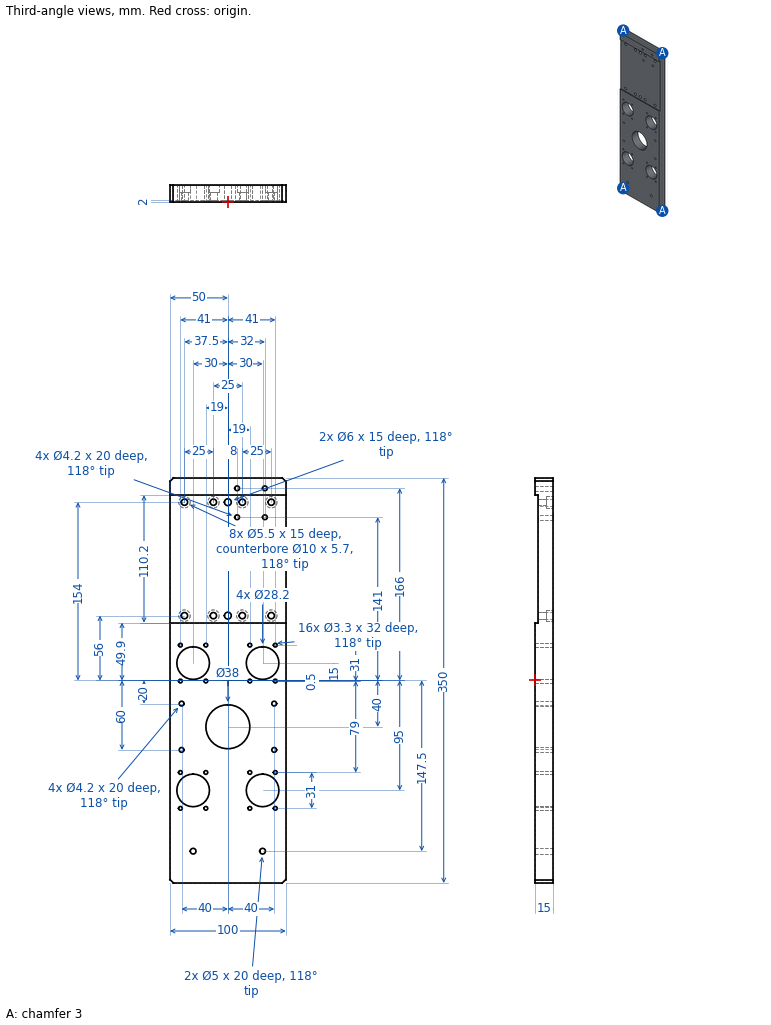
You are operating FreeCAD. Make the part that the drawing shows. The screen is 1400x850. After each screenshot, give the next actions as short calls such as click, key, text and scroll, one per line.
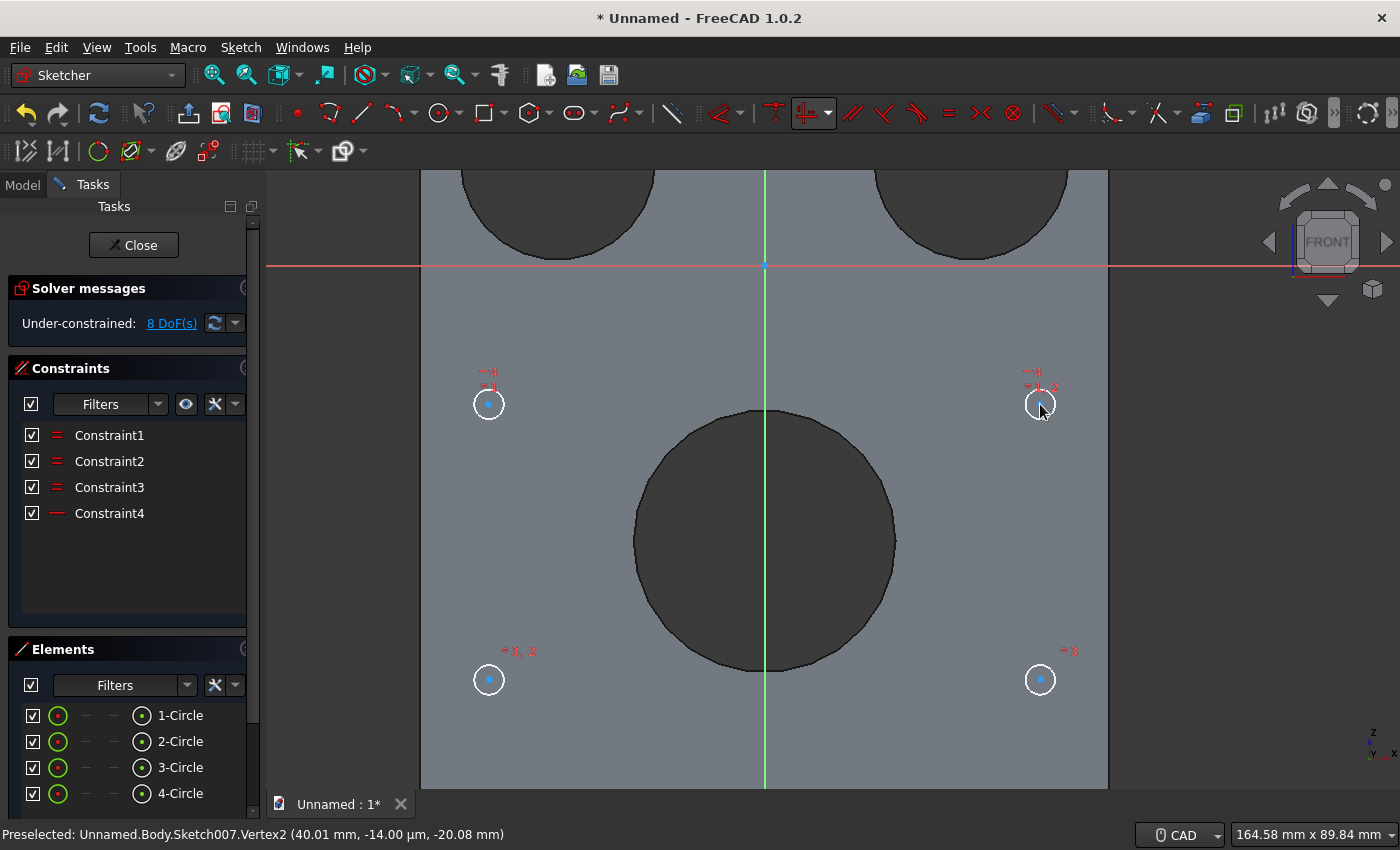
click(489, 404)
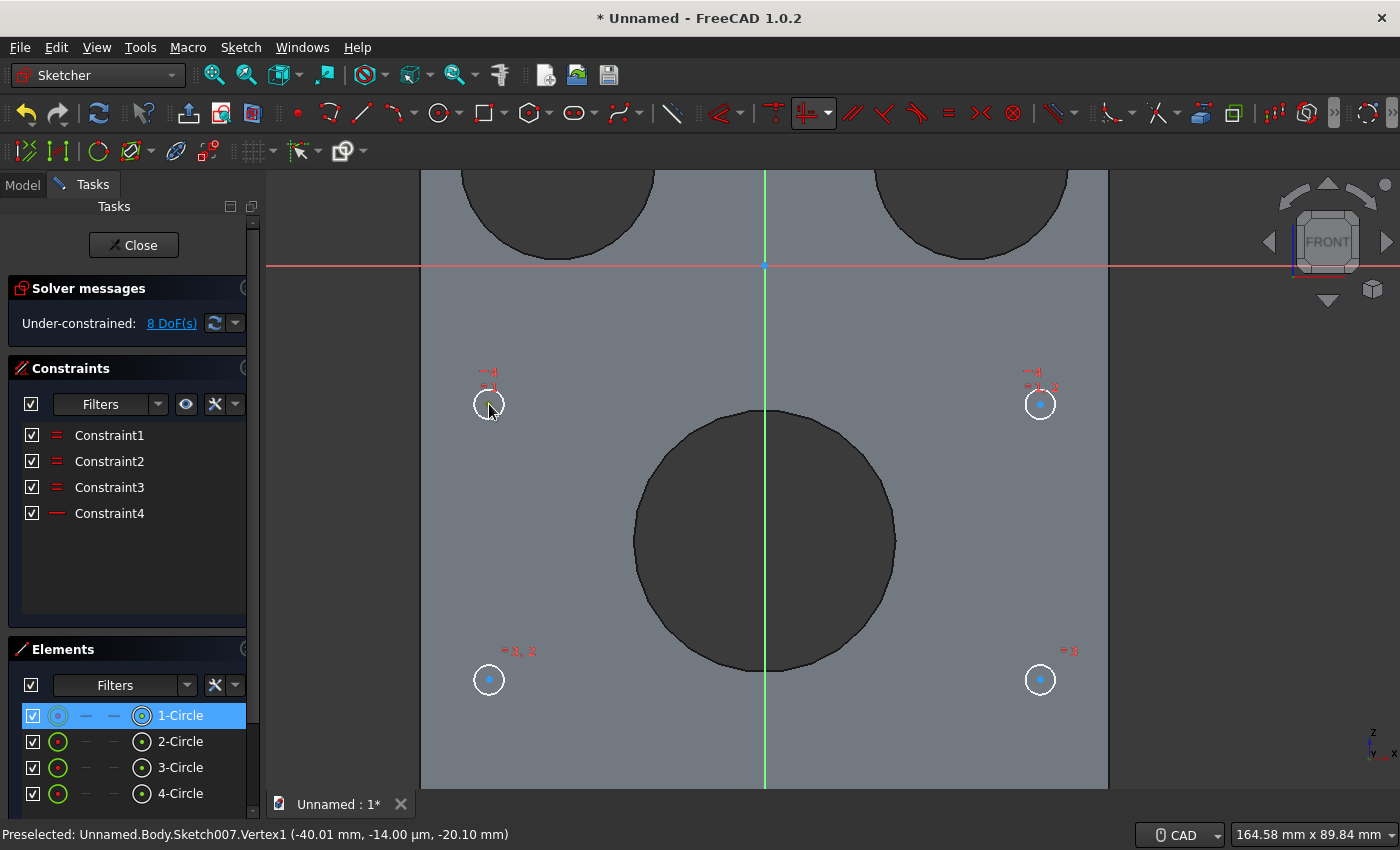
click(489, 680)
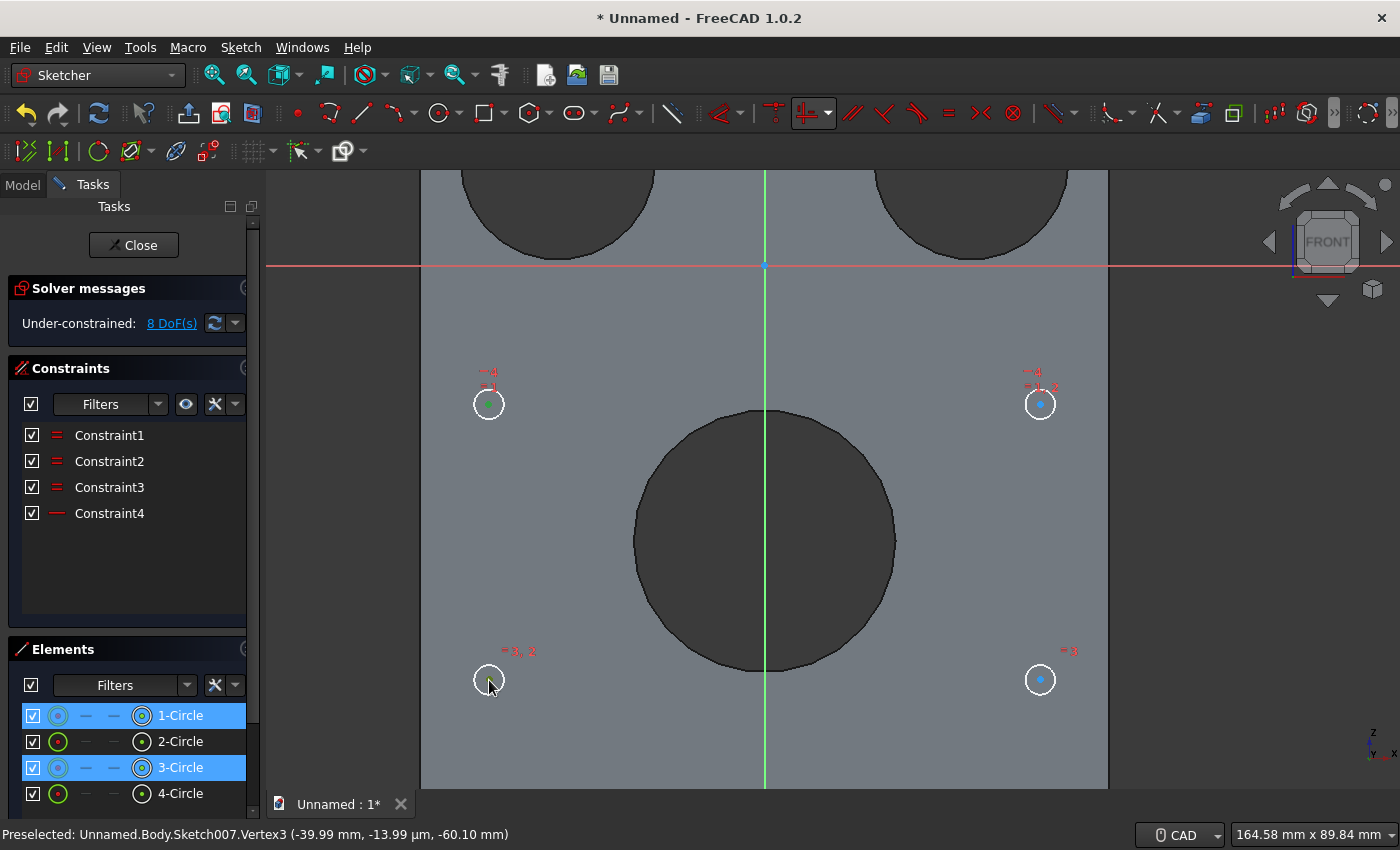
key(v)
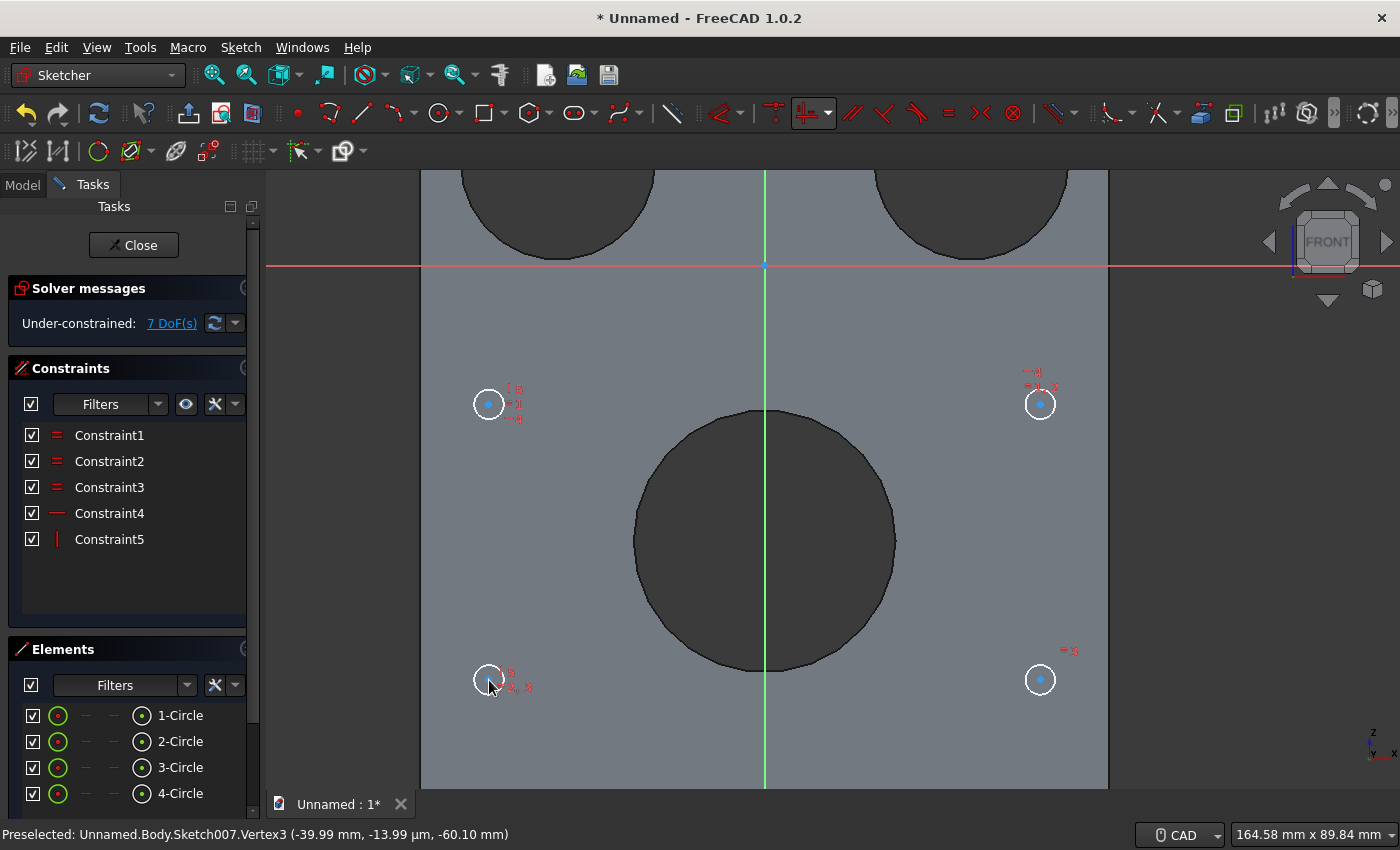
click(1040, 404)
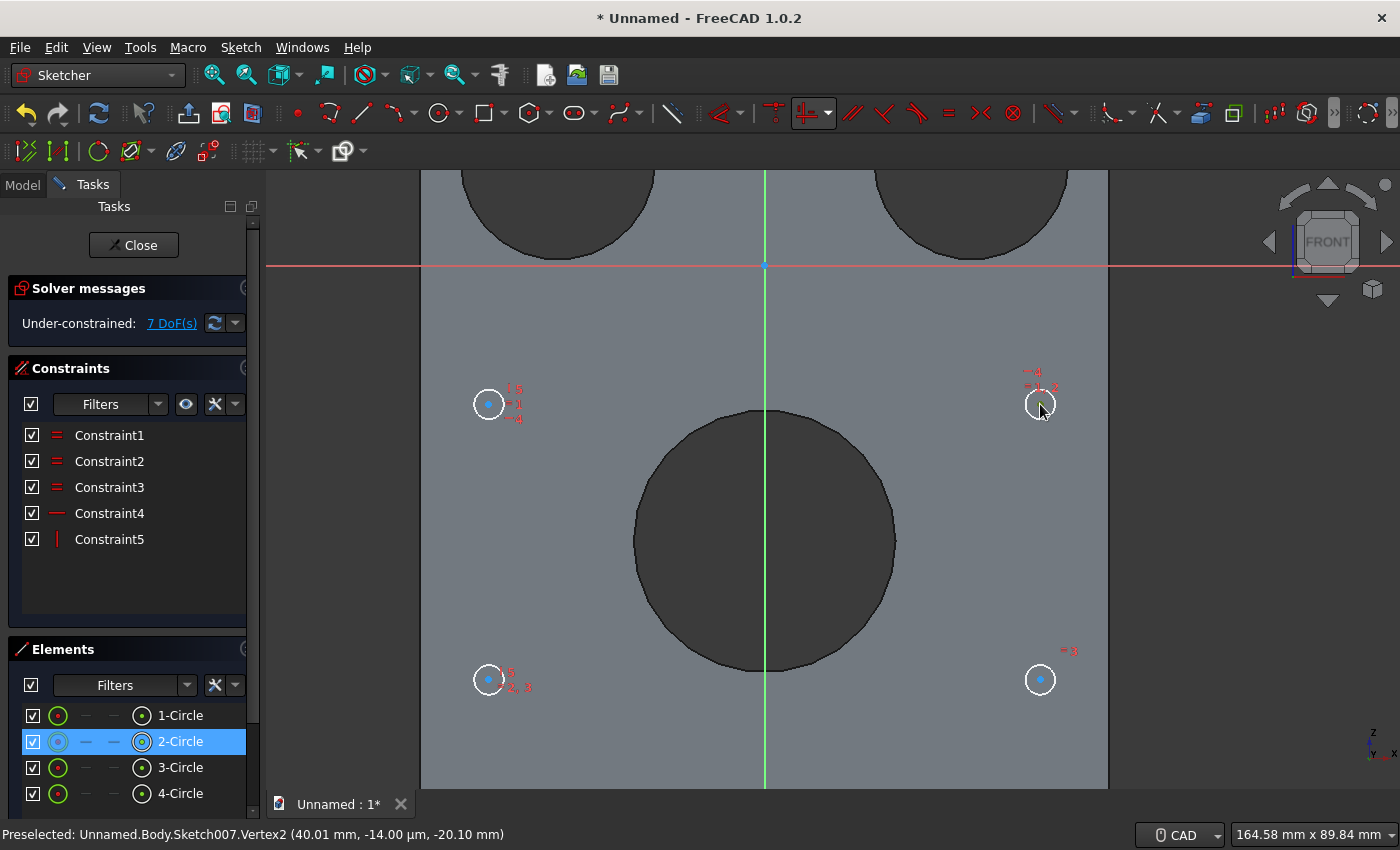
click(1040, 680)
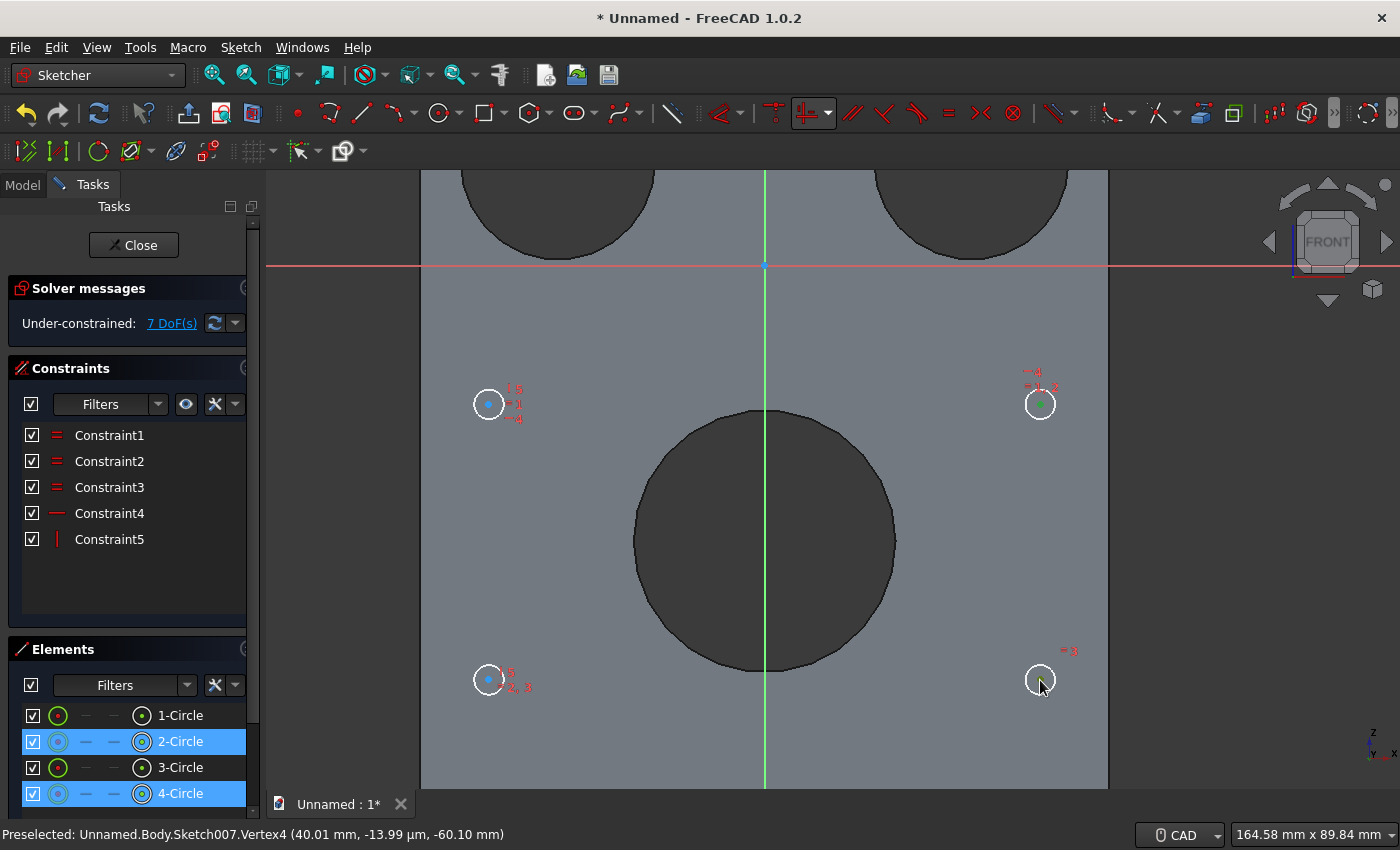
key(v)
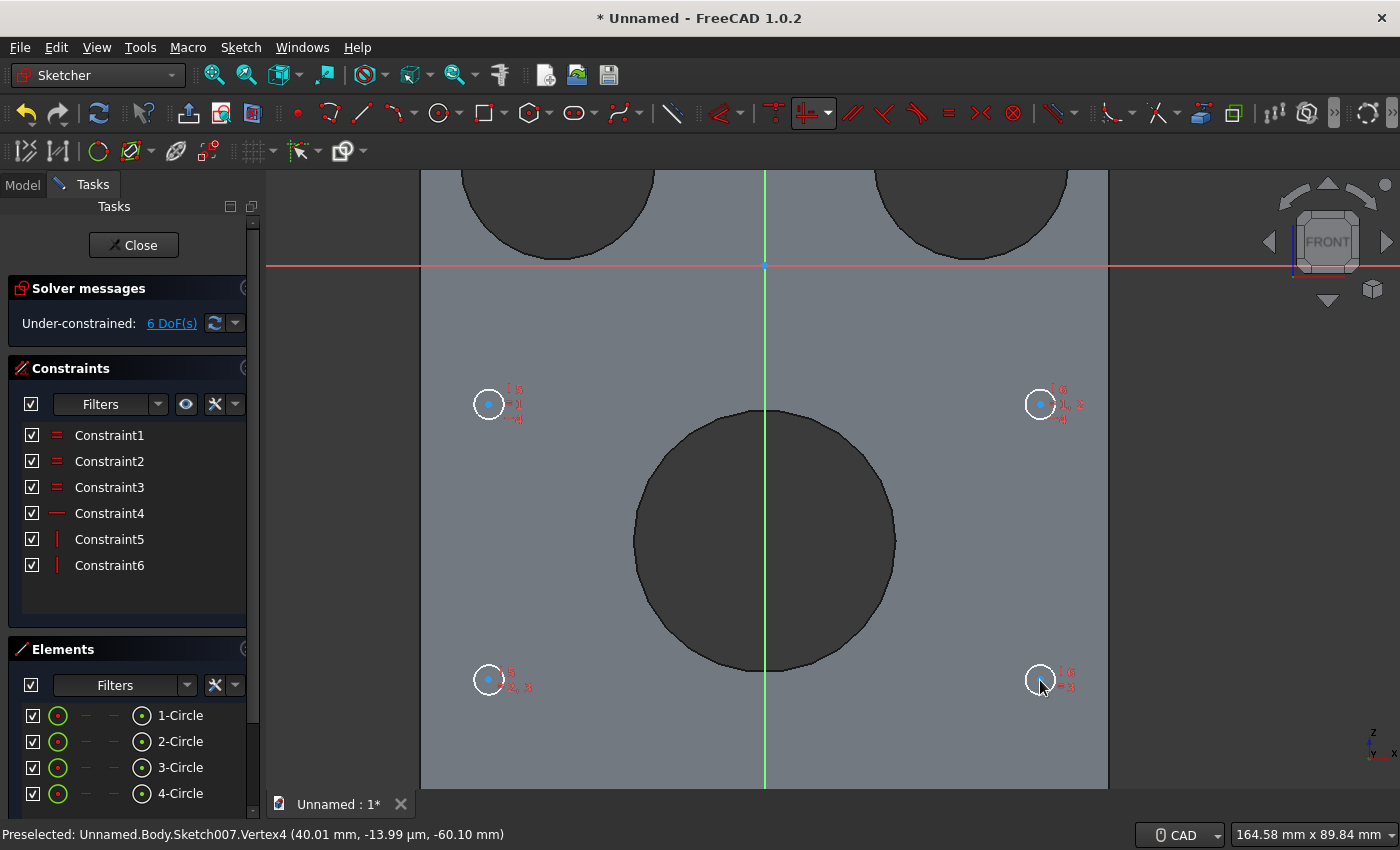
click(489, 680)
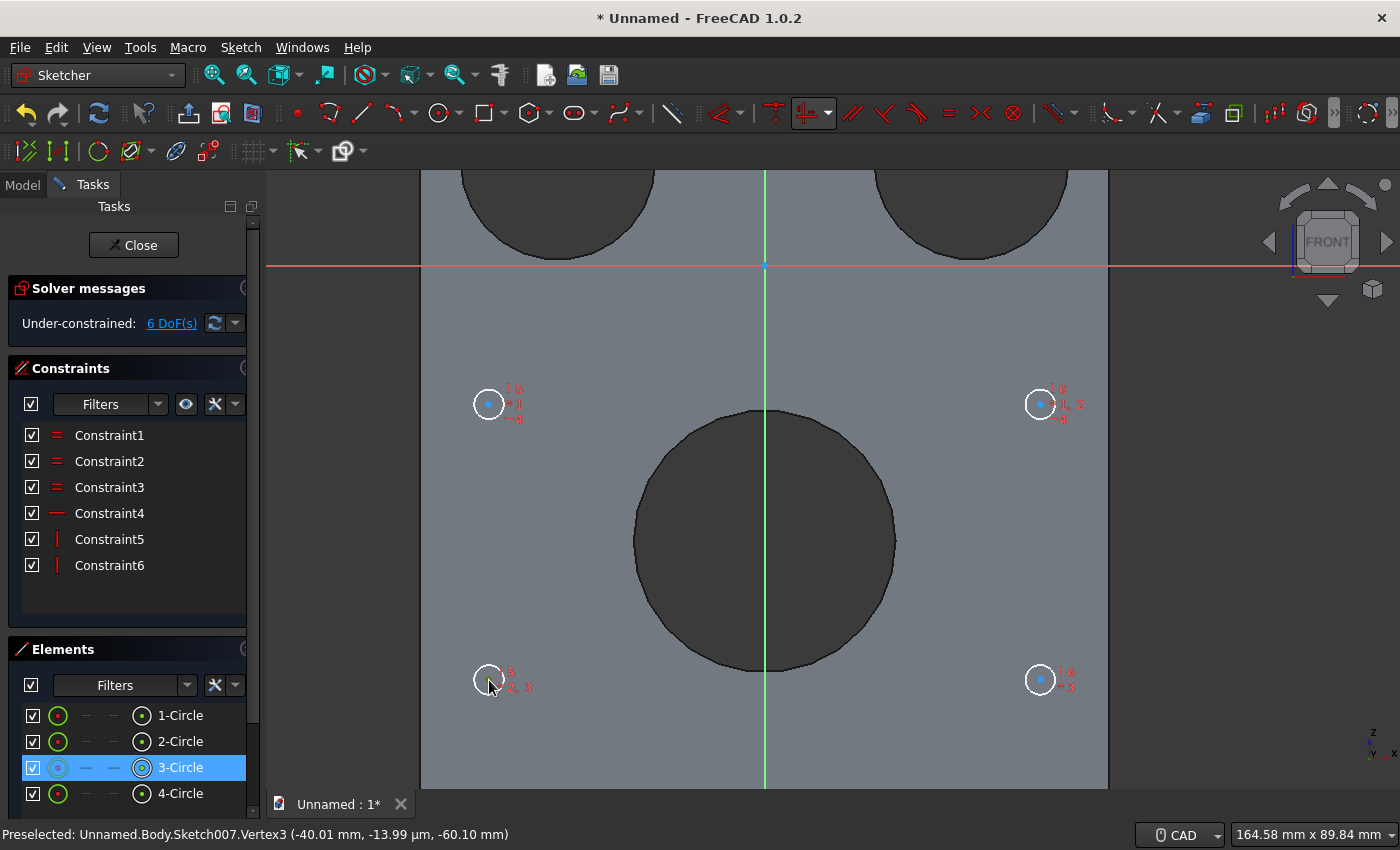
click(1040, 680)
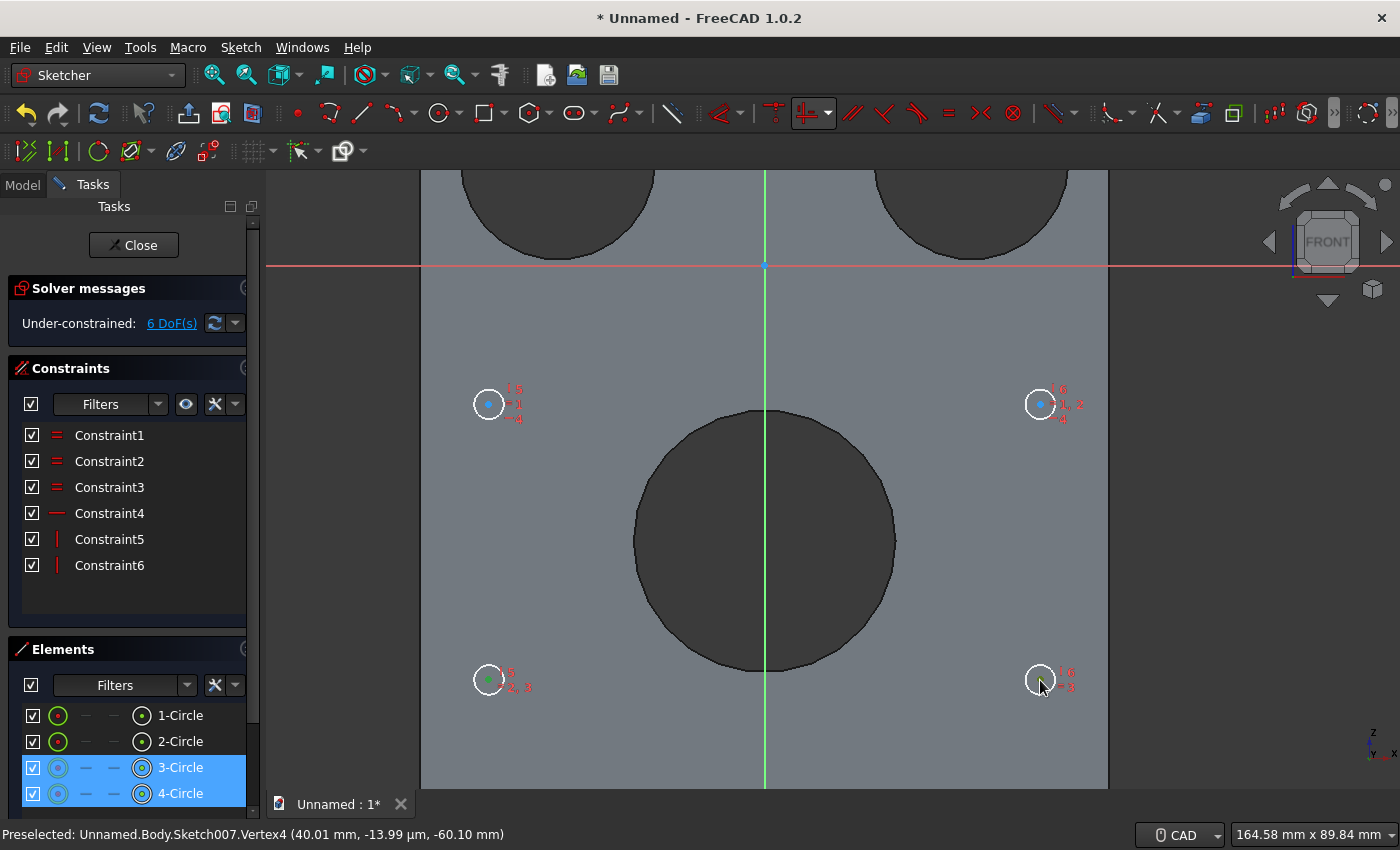
key(h)